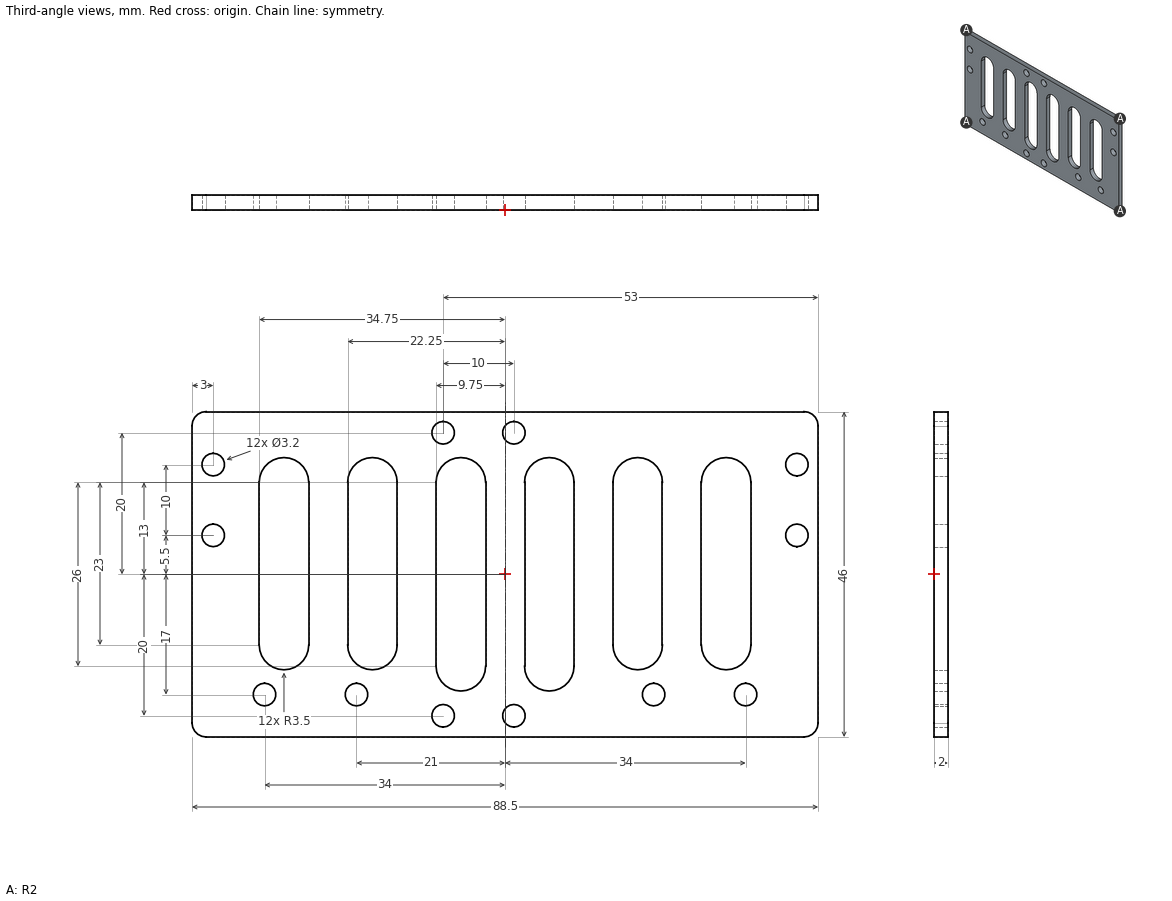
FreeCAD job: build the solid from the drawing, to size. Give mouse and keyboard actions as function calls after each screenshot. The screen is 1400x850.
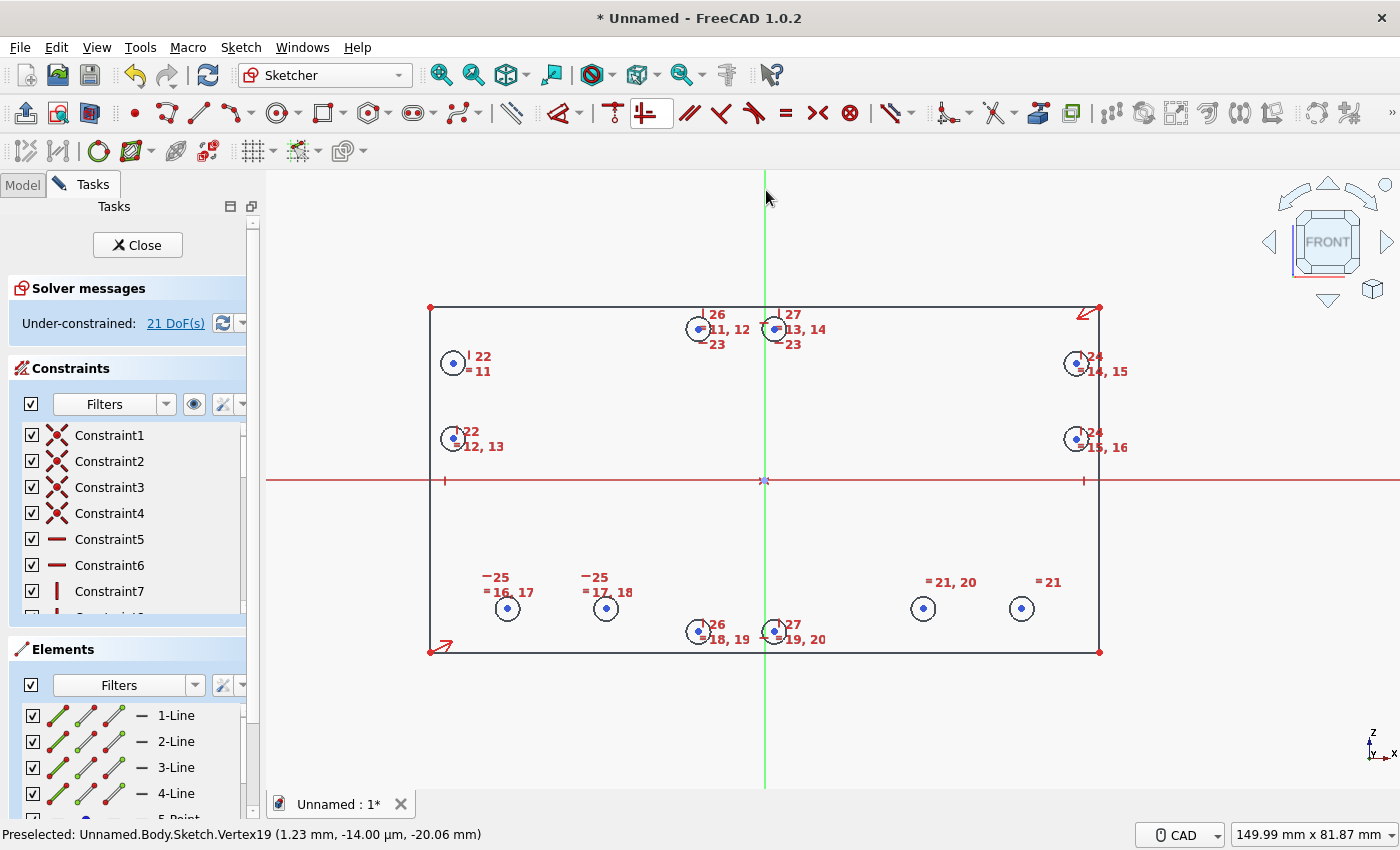
click(696, 634)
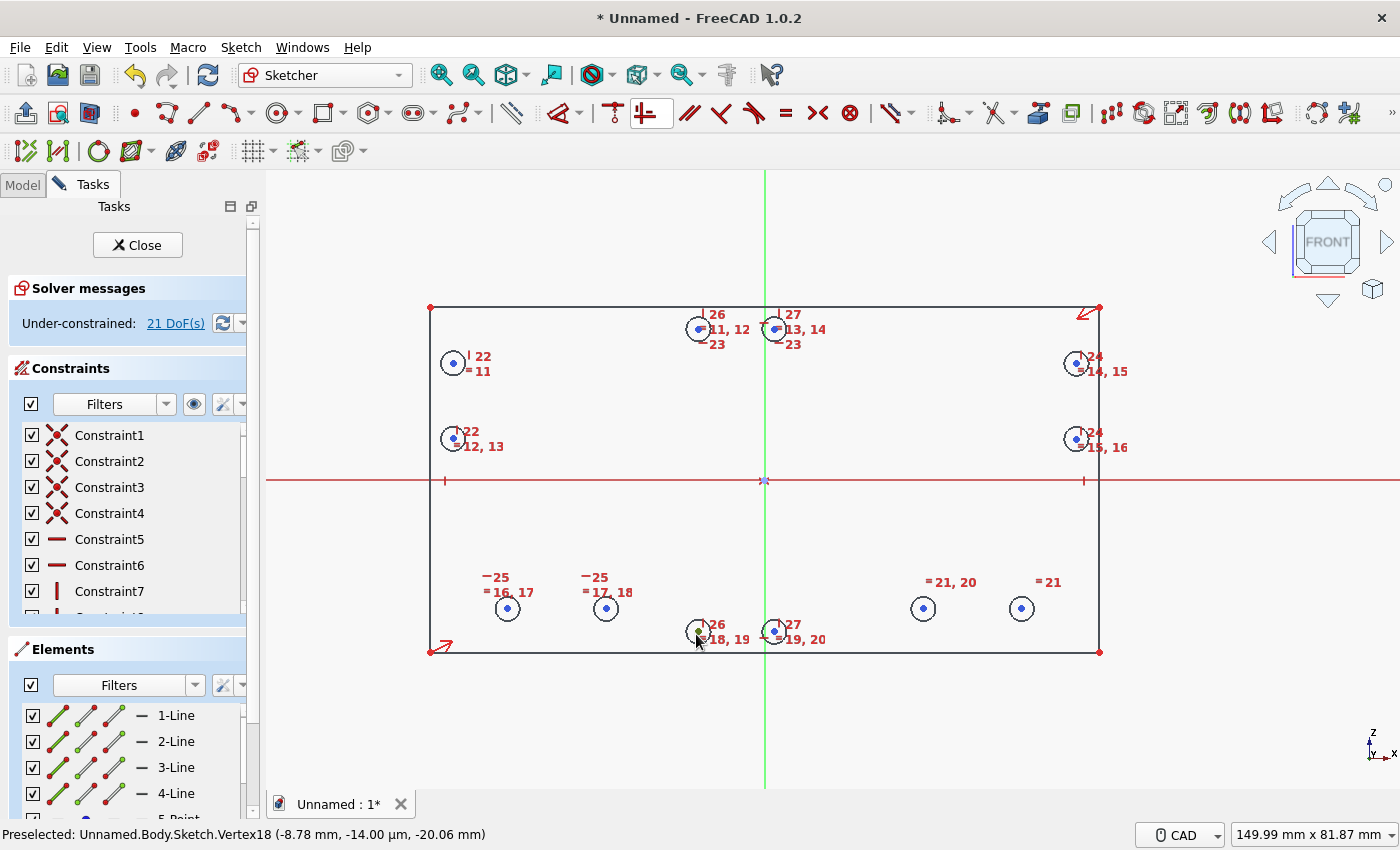
click(772, 634)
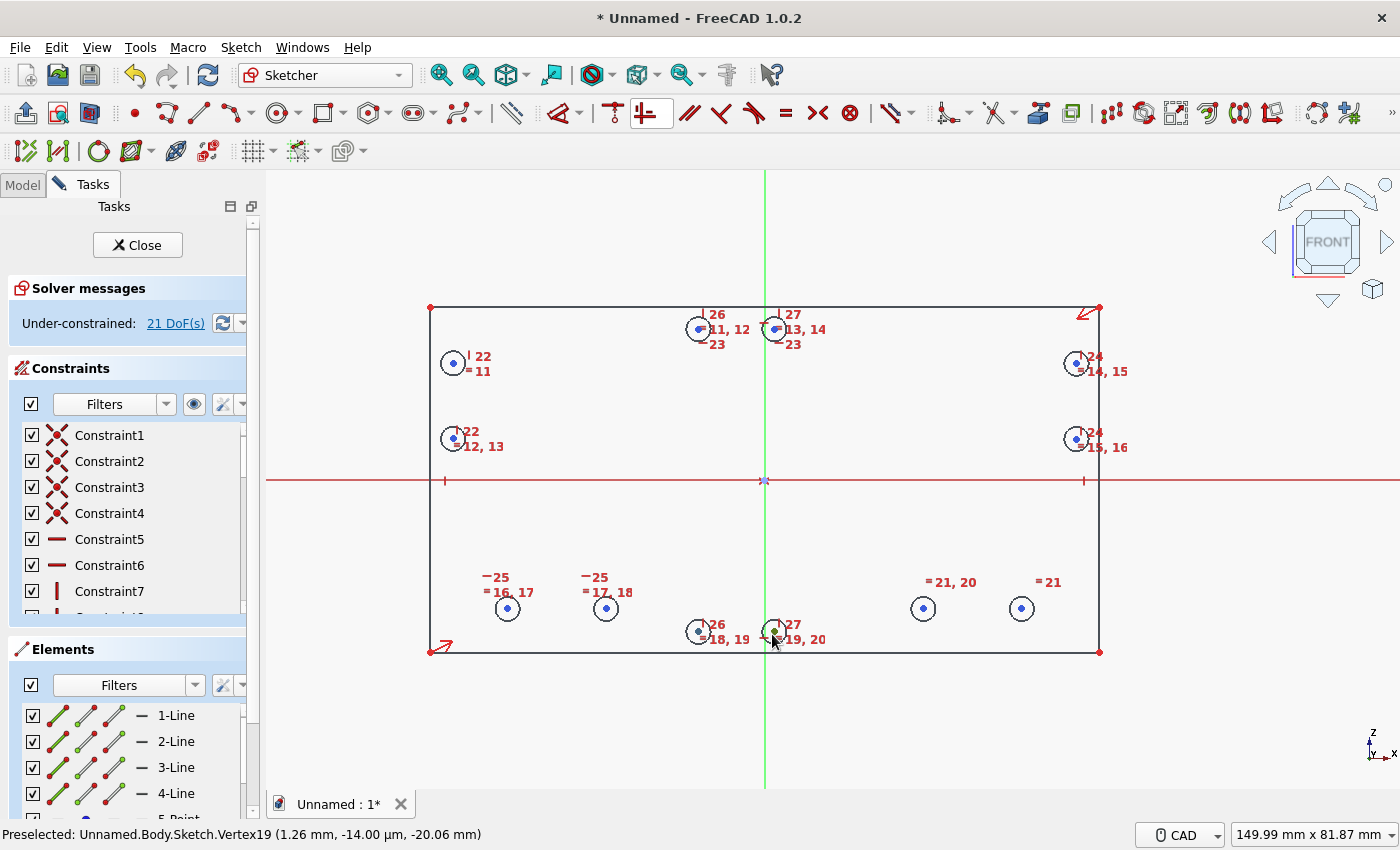
click(668, 114)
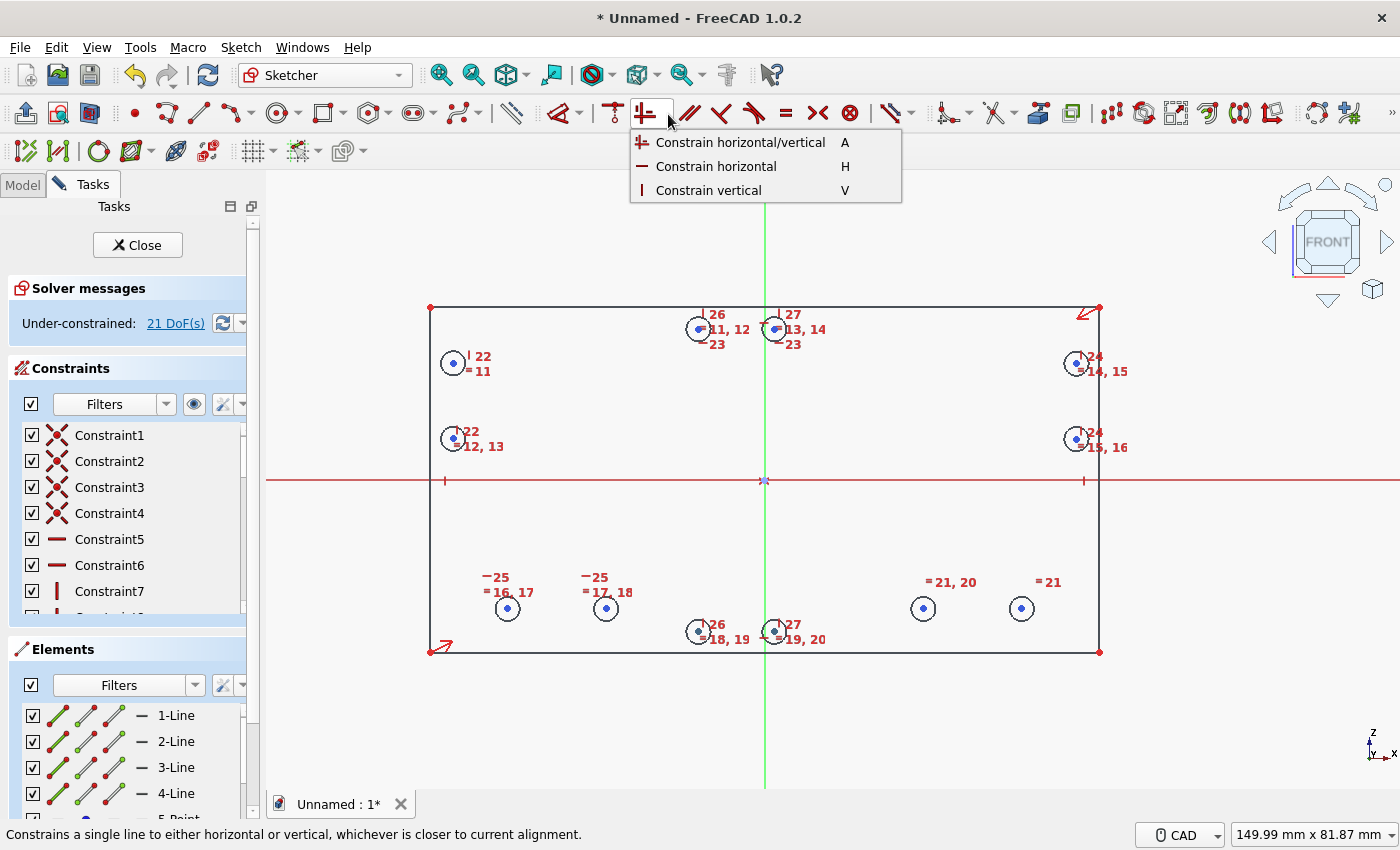
click(766, 166)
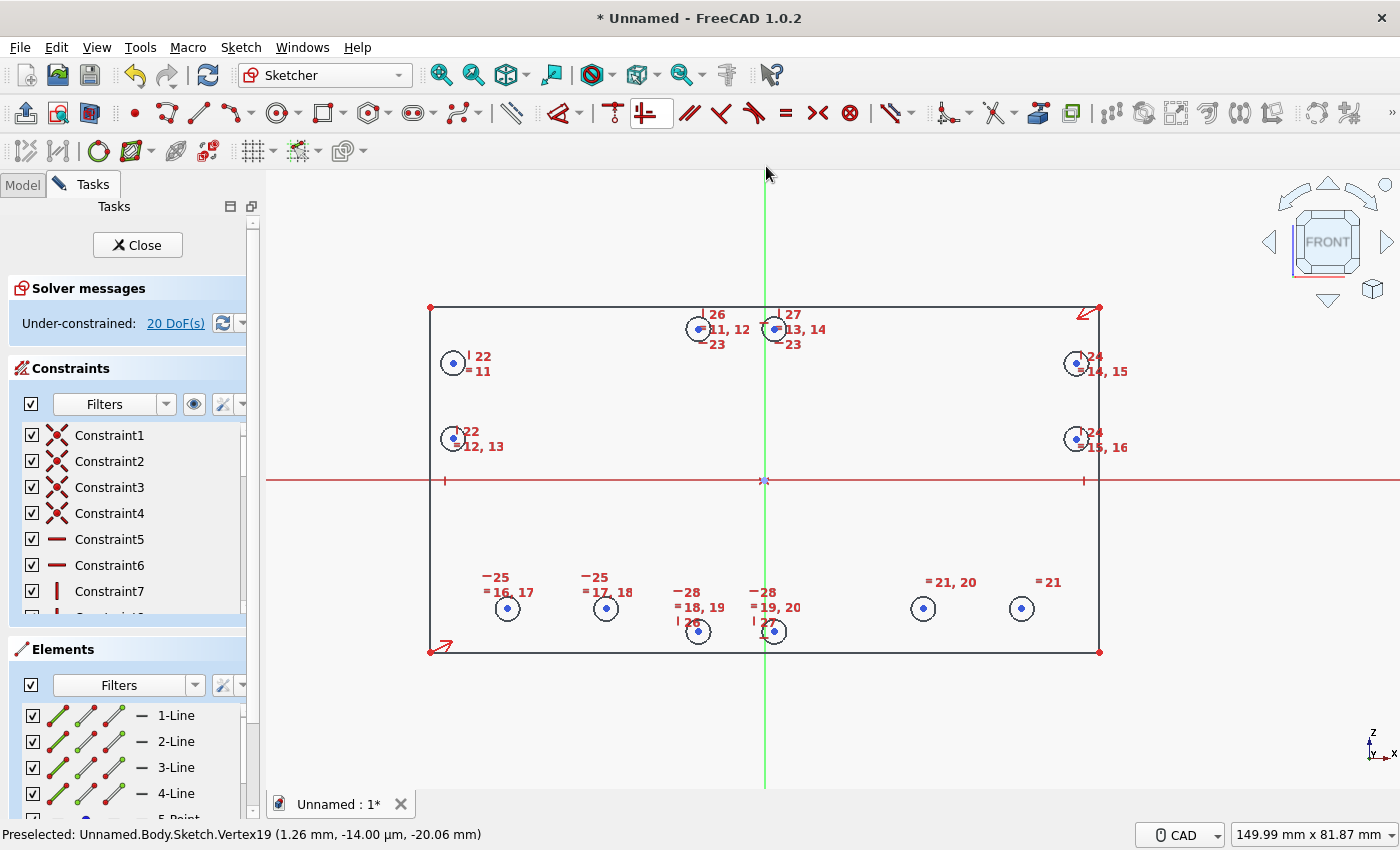
click(923, 609)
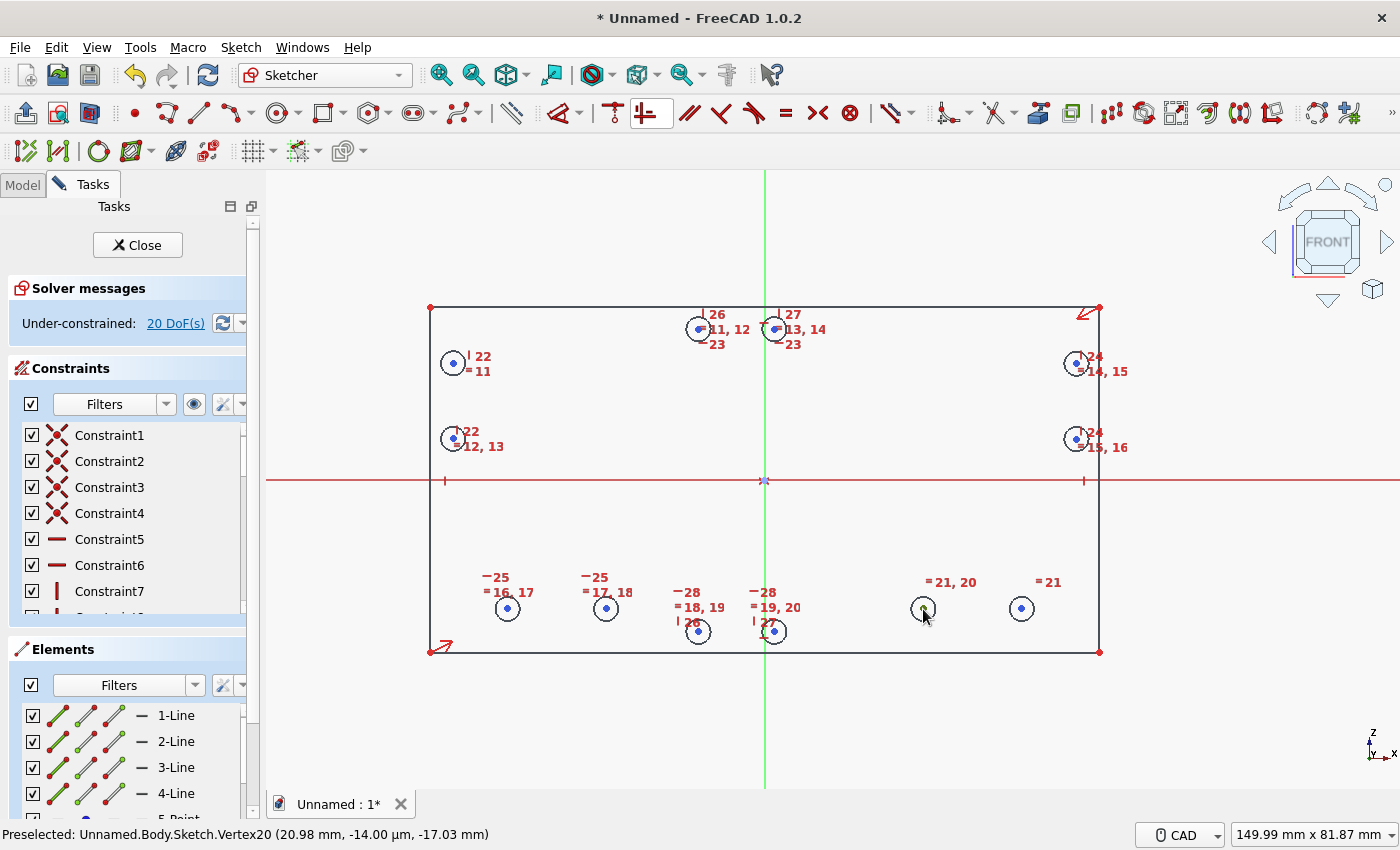
click(1022, 609)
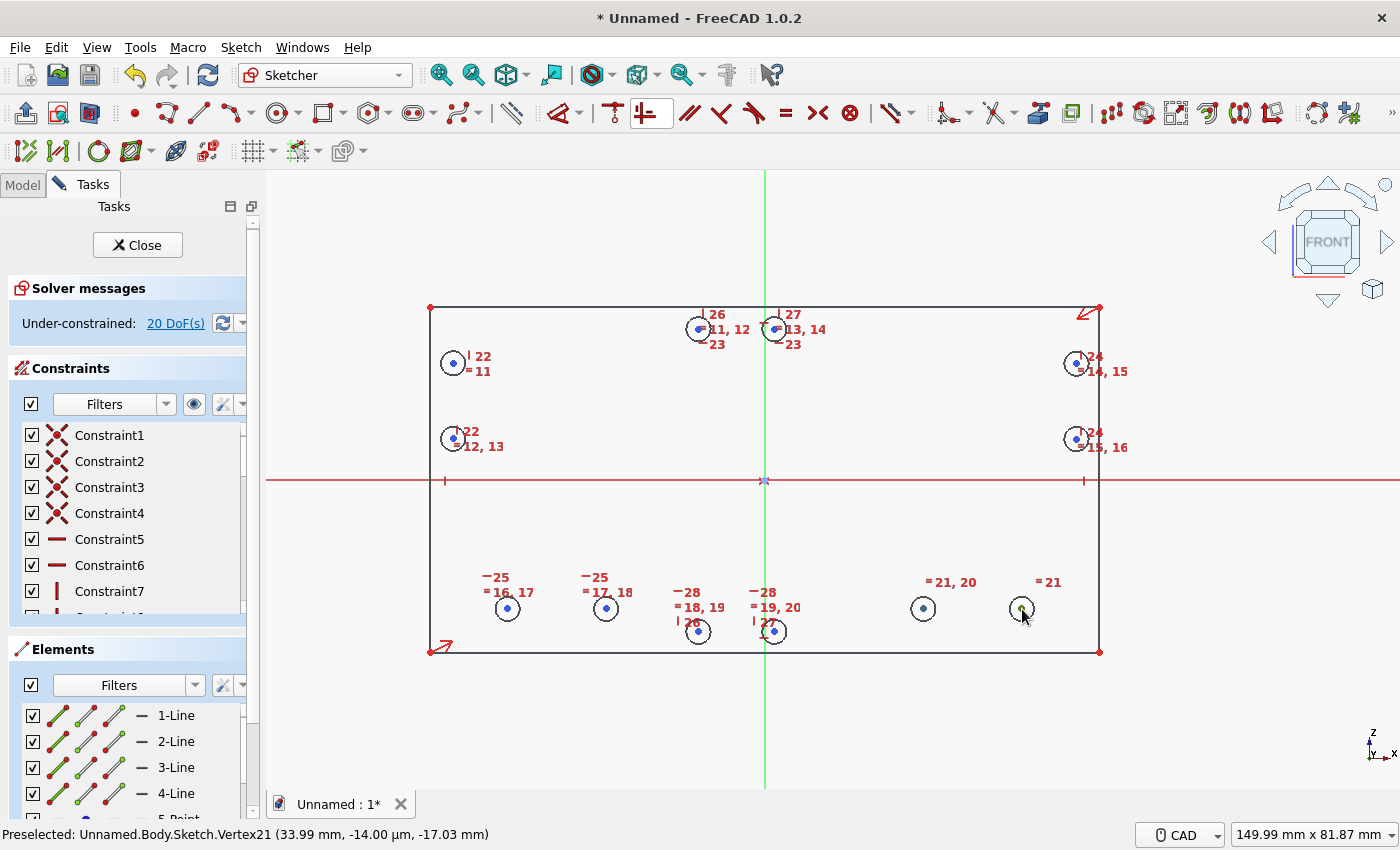
key(h)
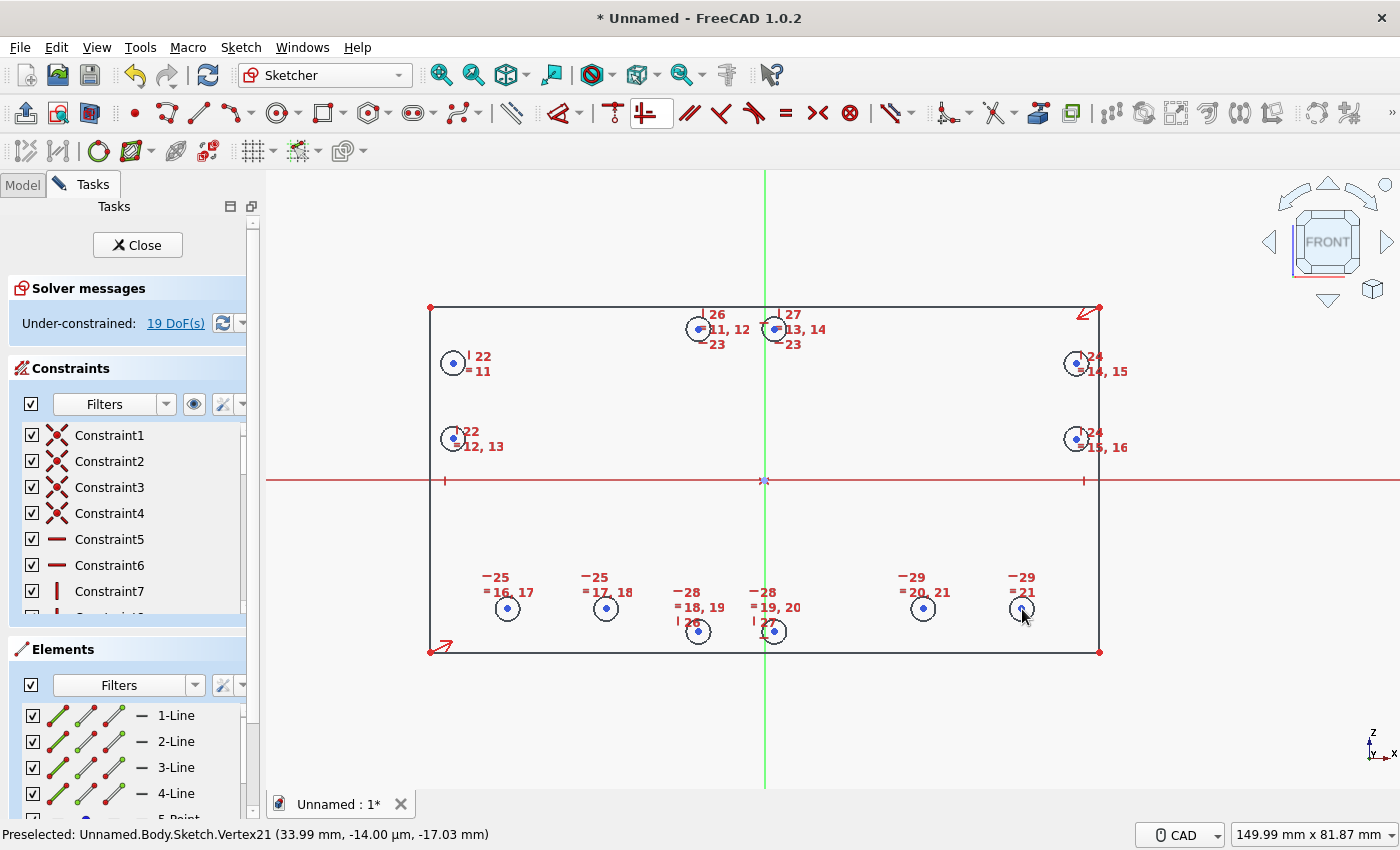
click(453, 363)